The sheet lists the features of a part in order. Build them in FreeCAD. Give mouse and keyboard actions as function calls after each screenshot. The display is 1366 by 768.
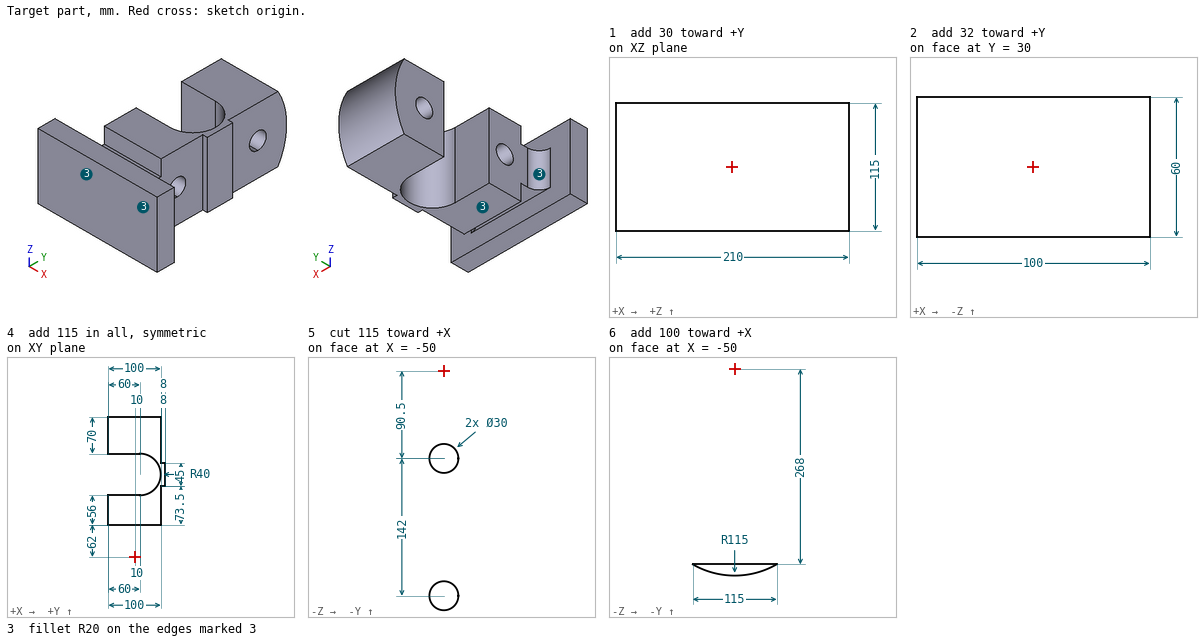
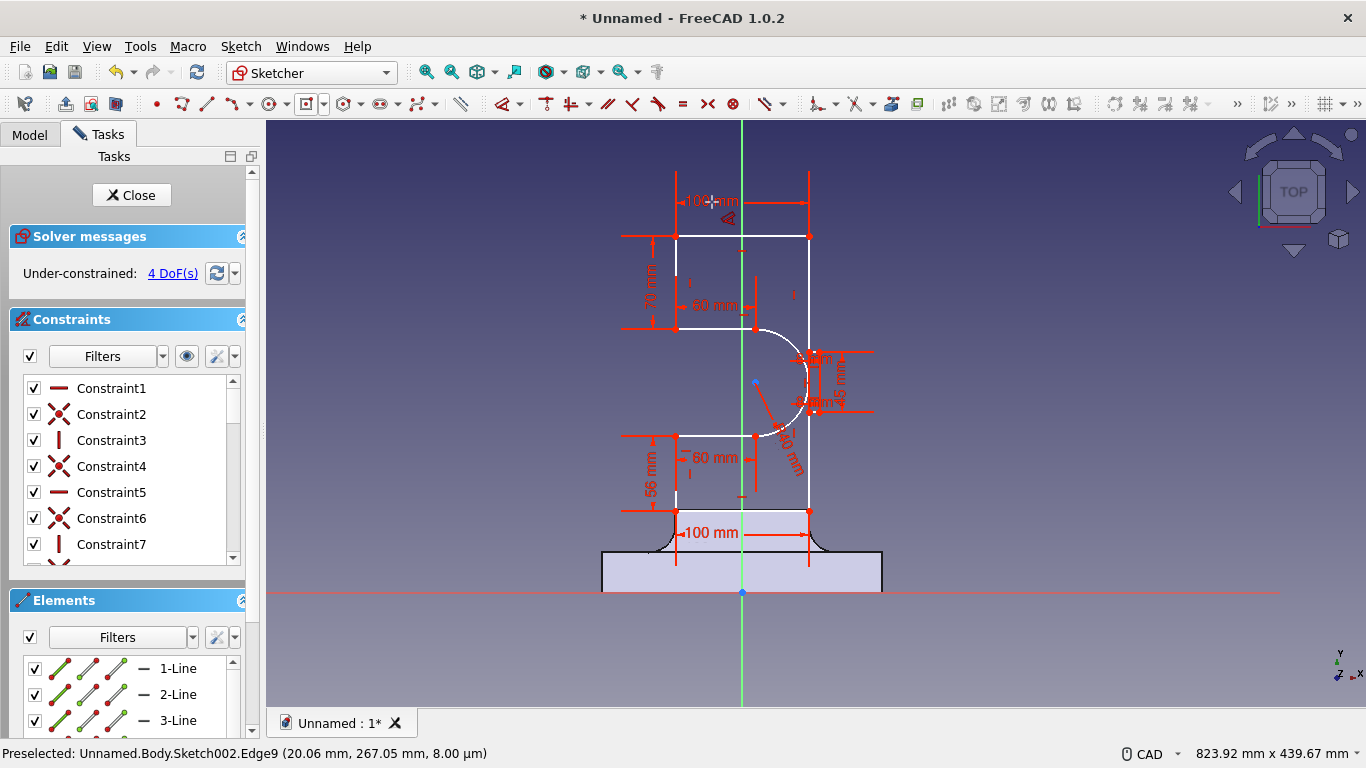
scroll(756, 436, up, 6)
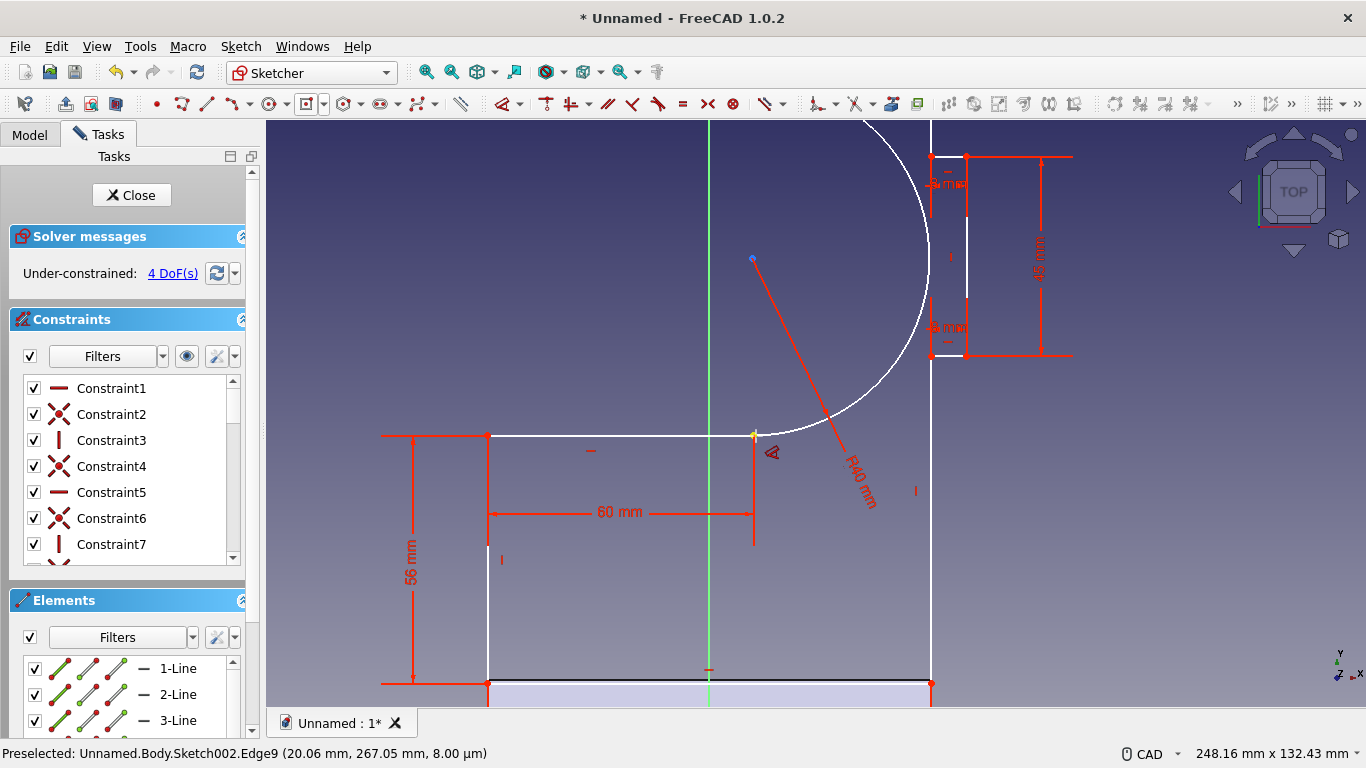
click(754, 436)
click(731, 402)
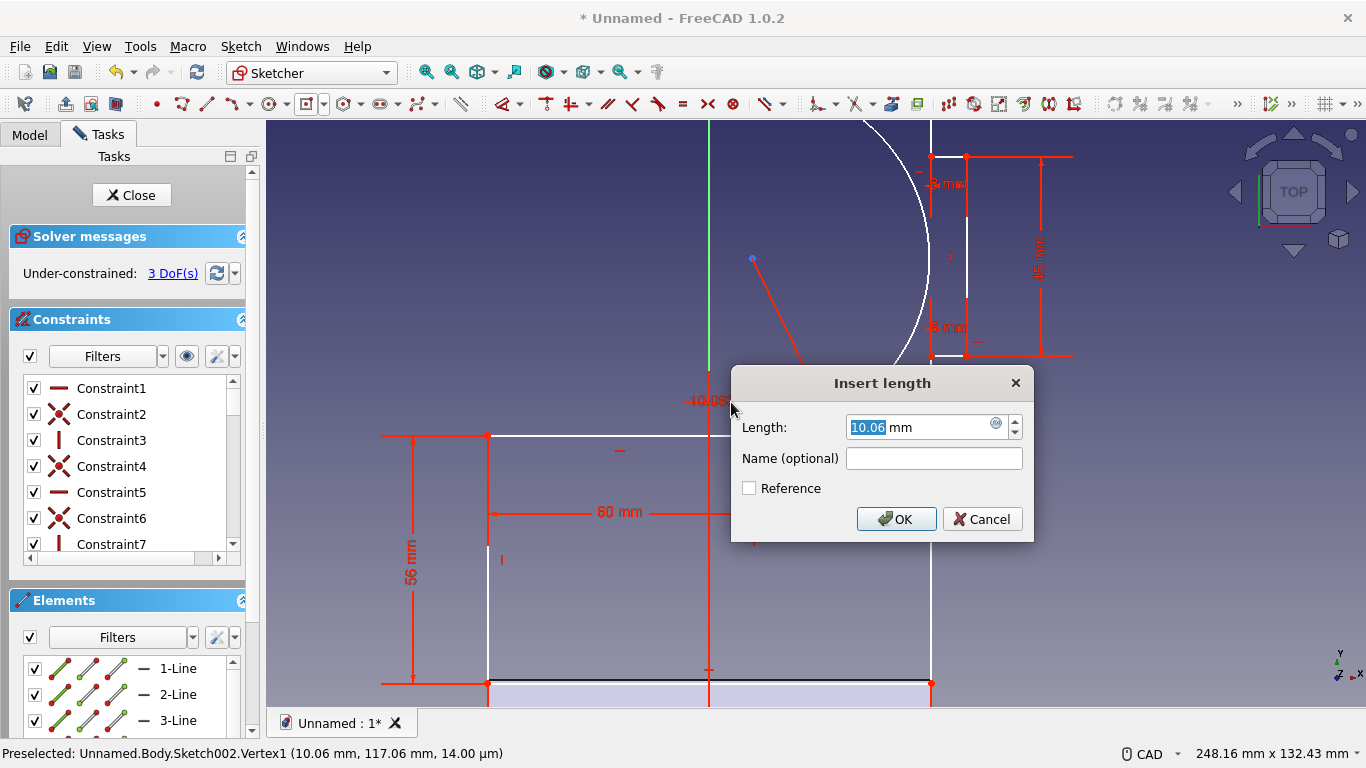
text(10)
key(Return)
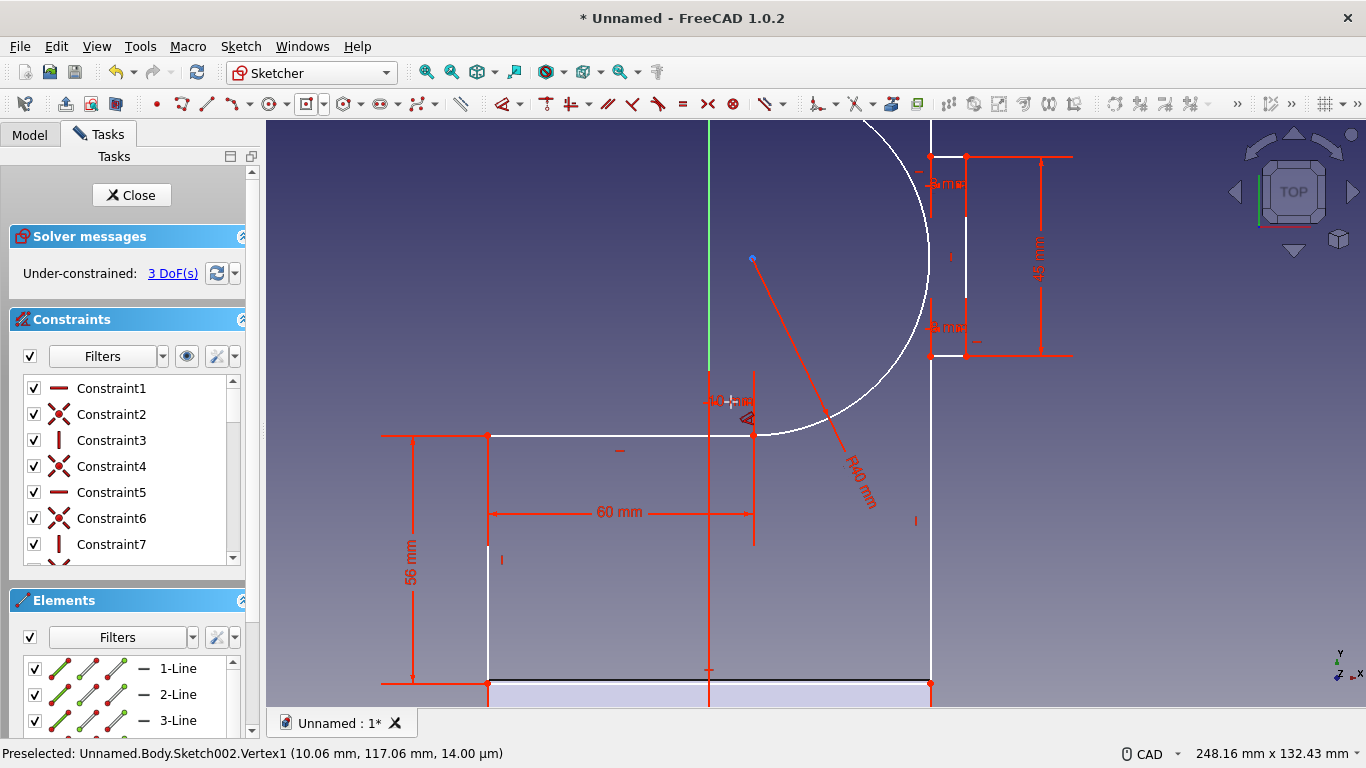
scroll(756, 436, down, 6)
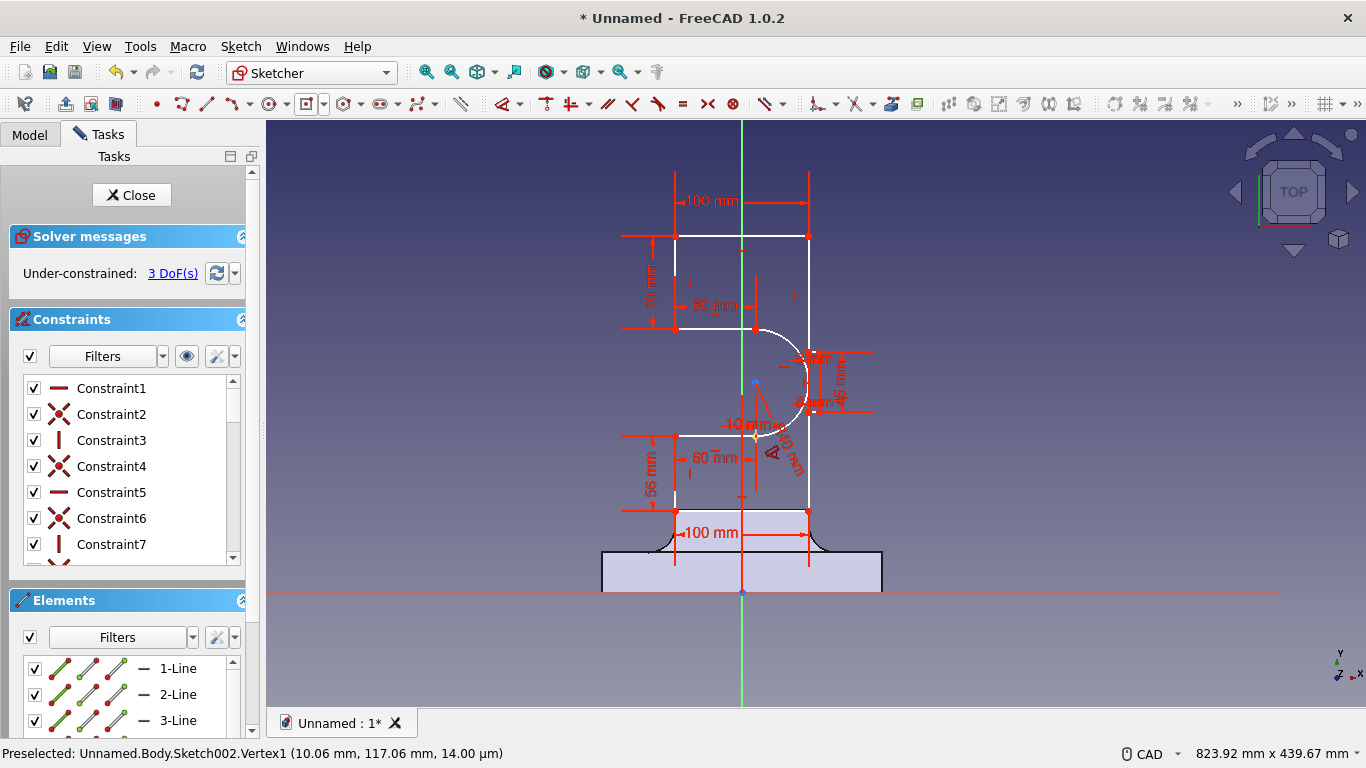
click(675, 511)
click(641, 552)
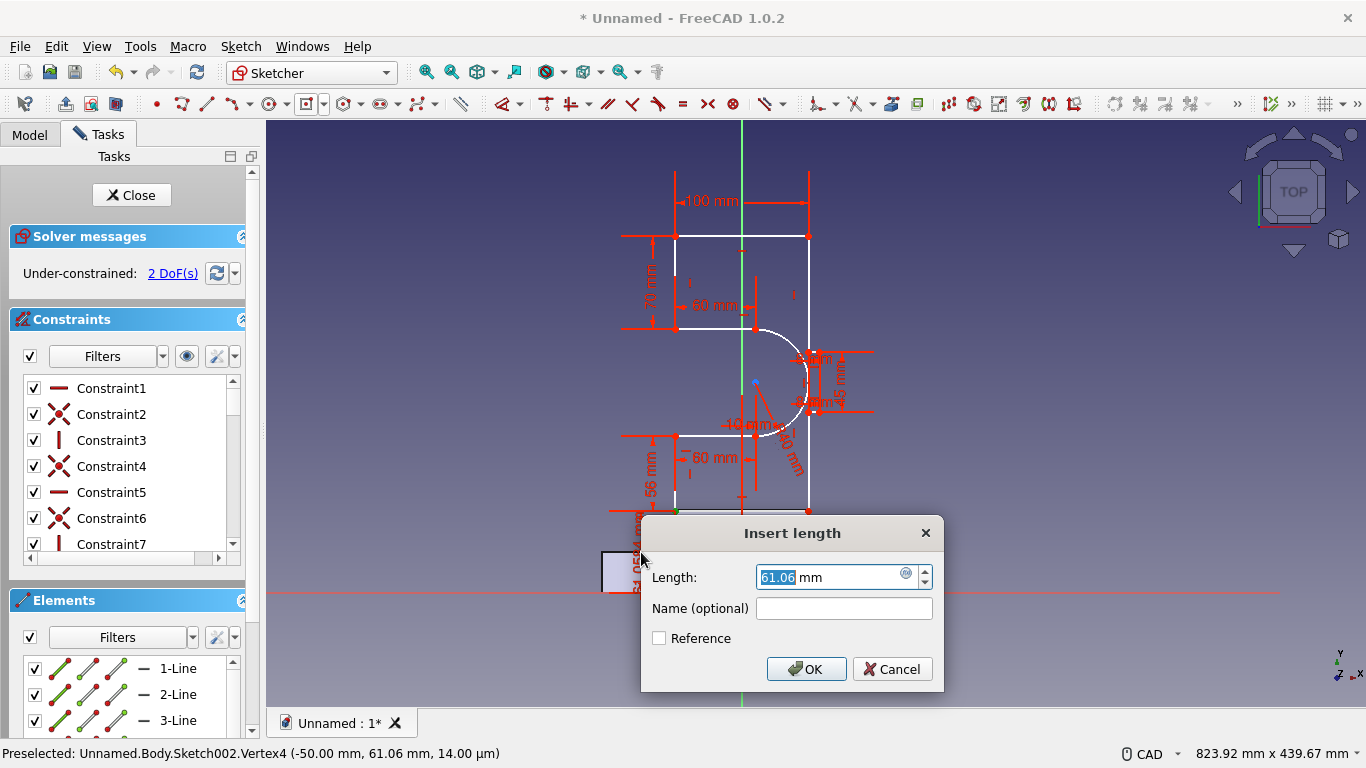
text(62)
key(Return)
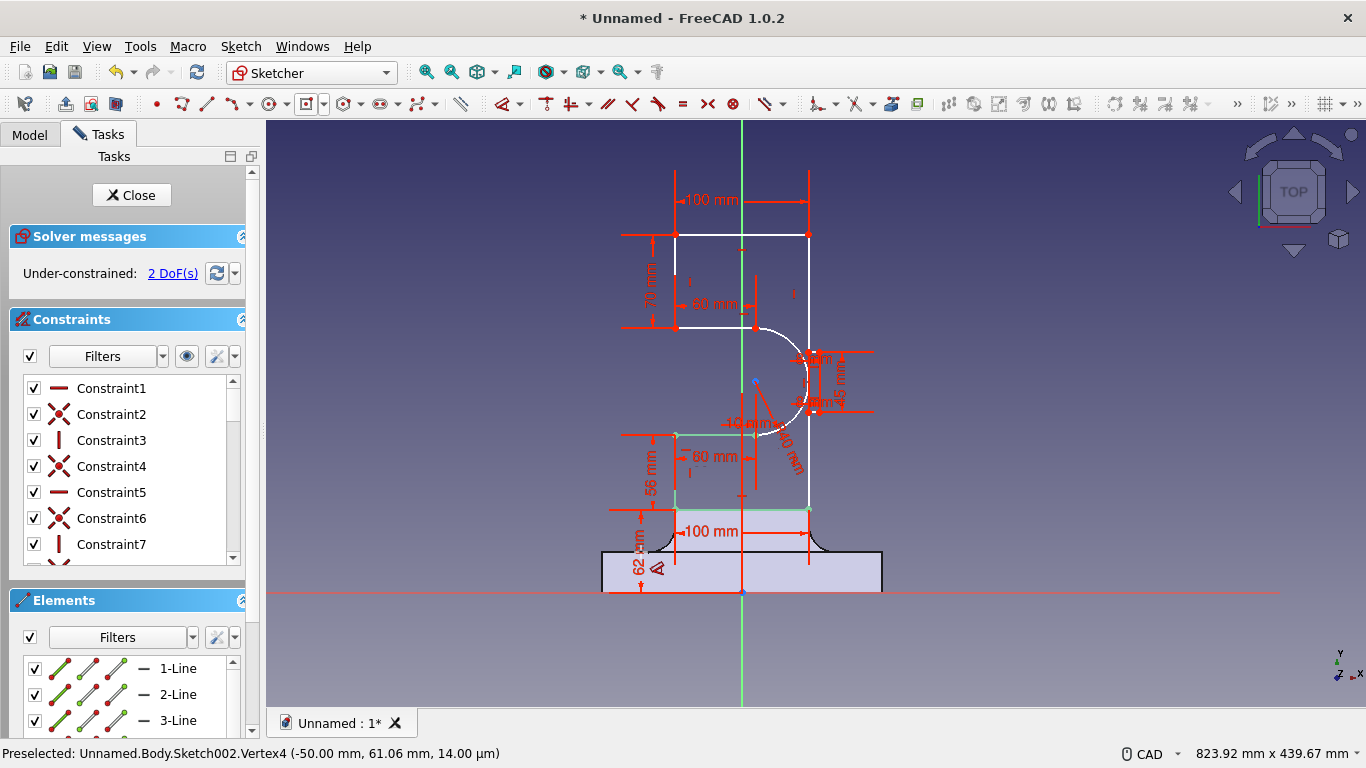
scroll(755, 382, up, 6)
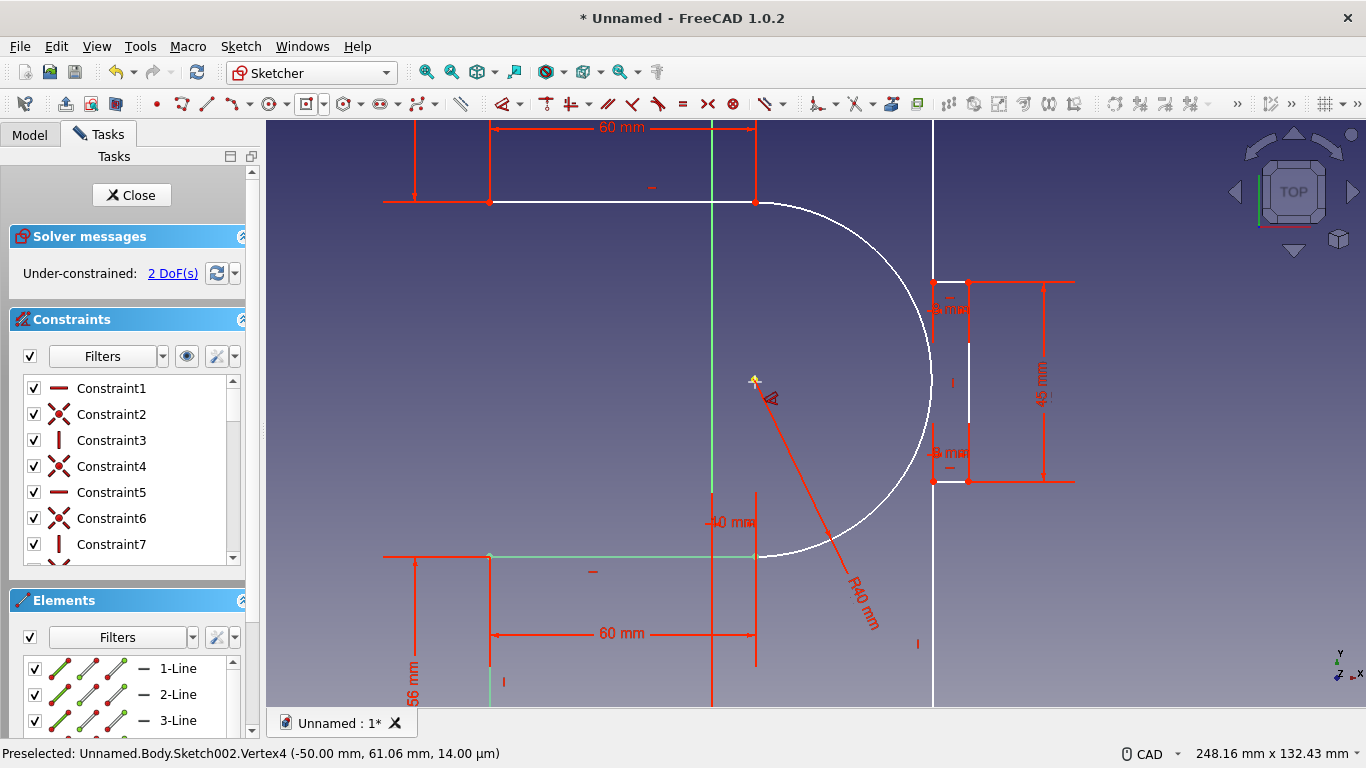
click(754, 380)
click(733, 346)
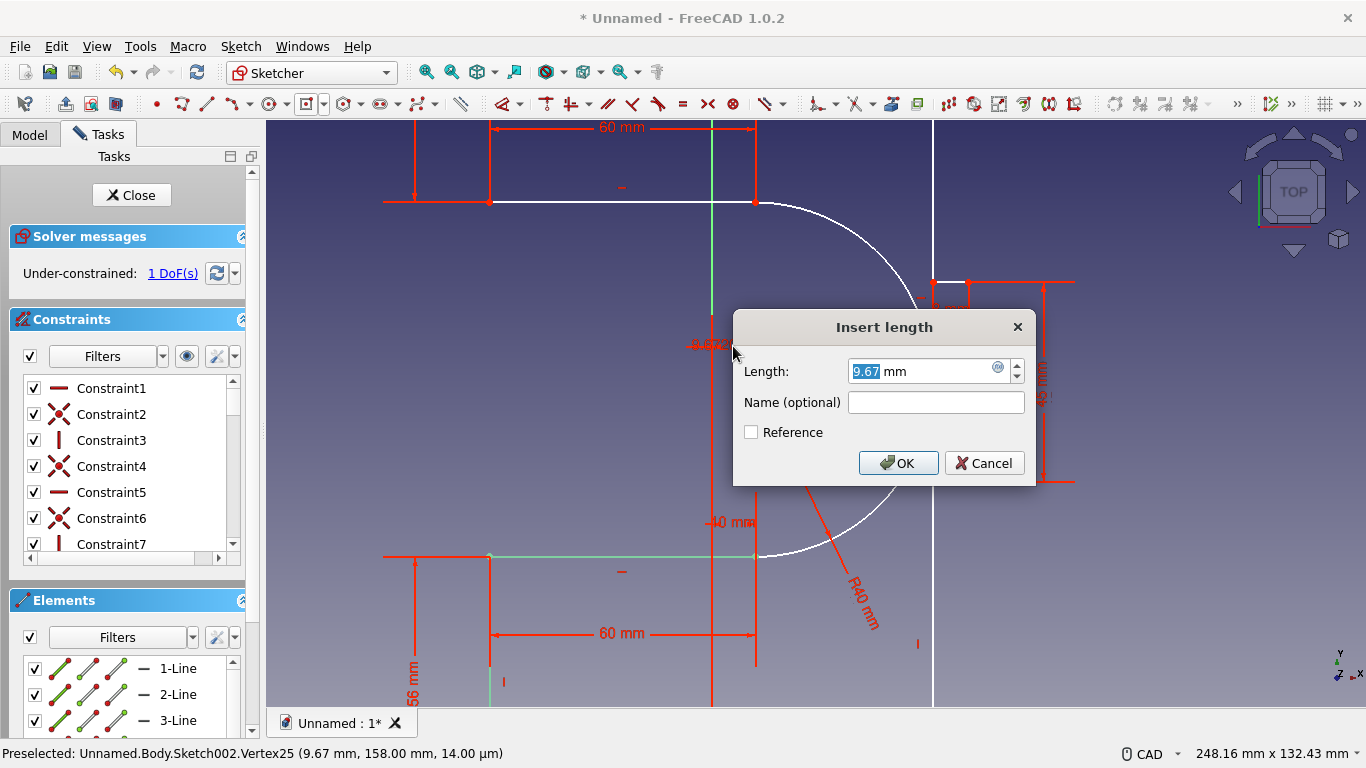
text(10)
key(Return)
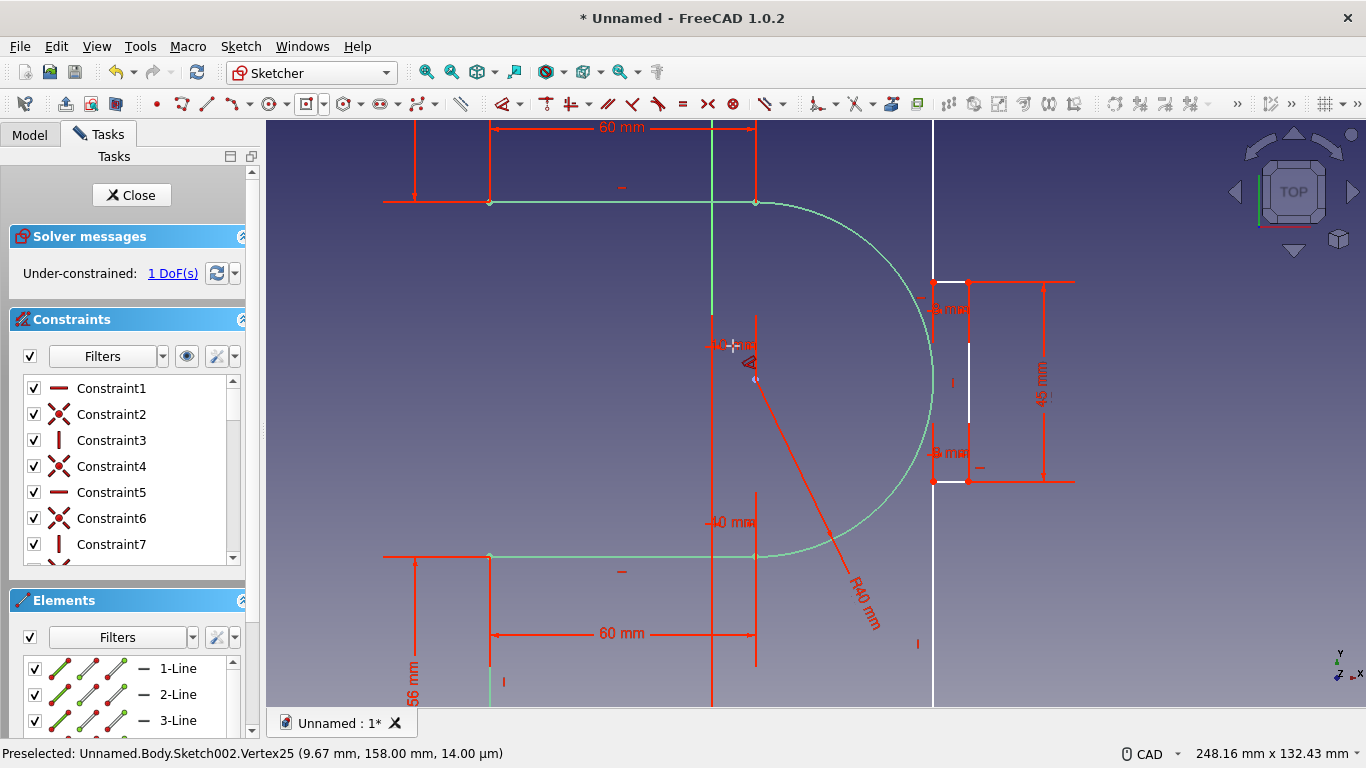
click(933, 579)
click(967, 580)